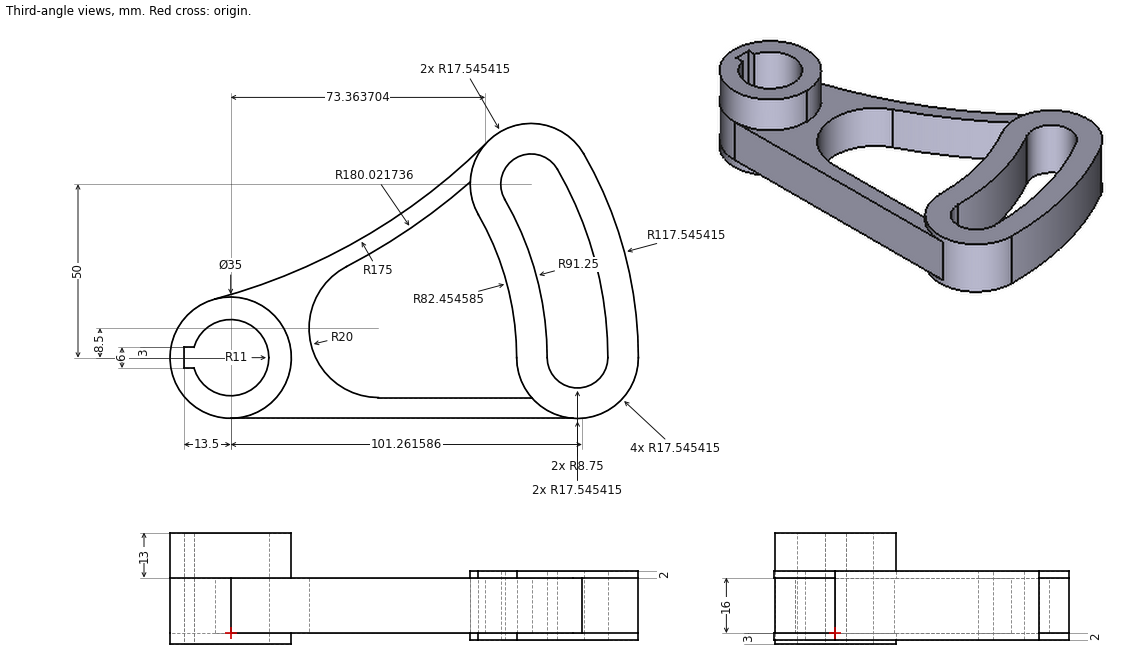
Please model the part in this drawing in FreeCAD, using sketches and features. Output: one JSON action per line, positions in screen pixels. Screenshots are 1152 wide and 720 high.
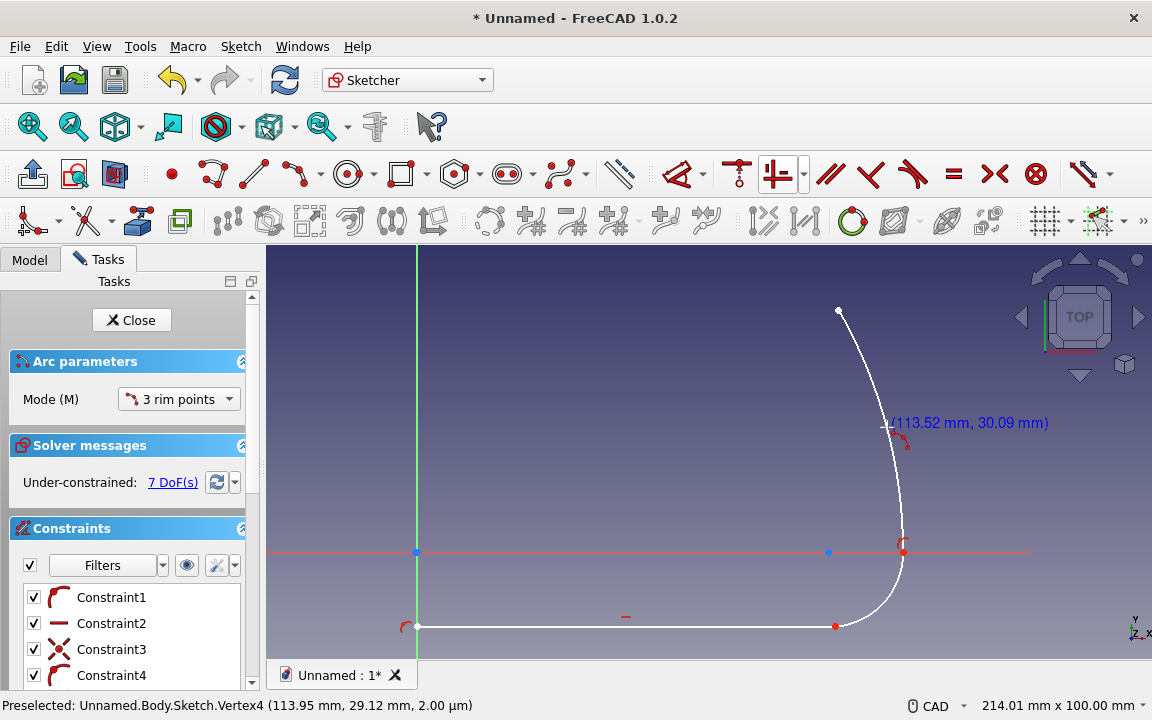
{"action": "left_click", "coordinate": [839, 310]}
{"action": "left_click", "coordinate": [721, 298]}
{"action": "left_click", "coordinate": [783, 273]}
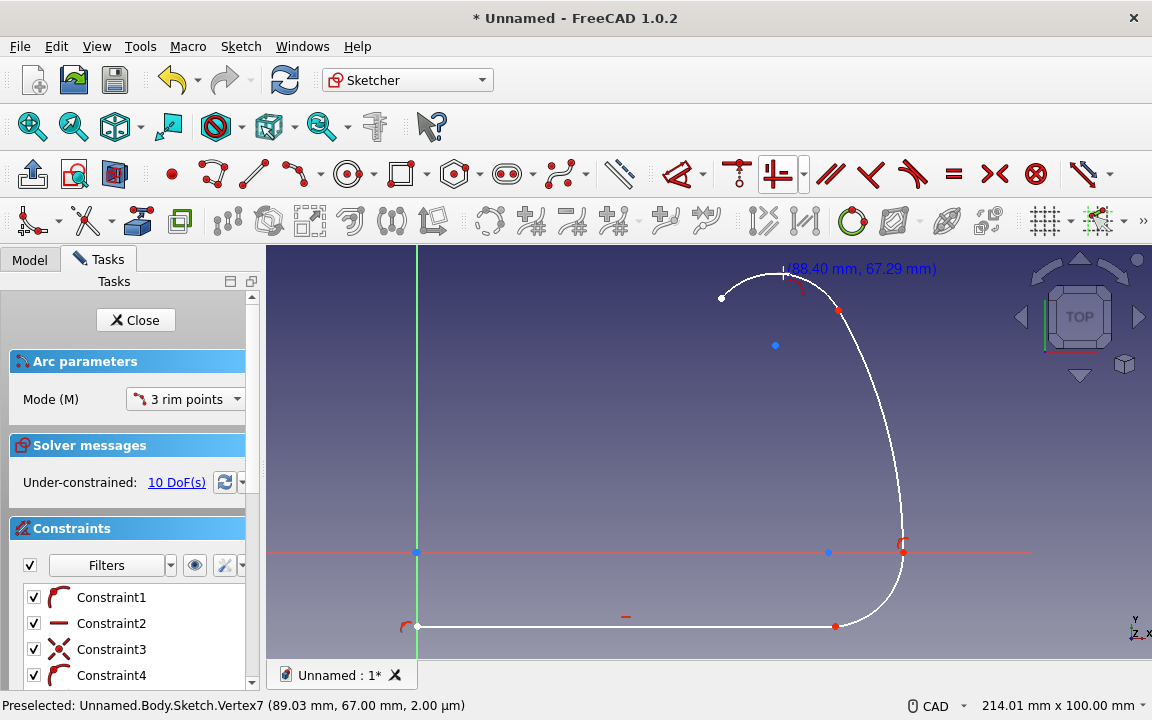
{"action": "left_click", "coordinate": [721, 299]}
{"action": "left_click", "coordinate": [398, 483]}
{"action": "left_click", "coordinate": [572, 411]}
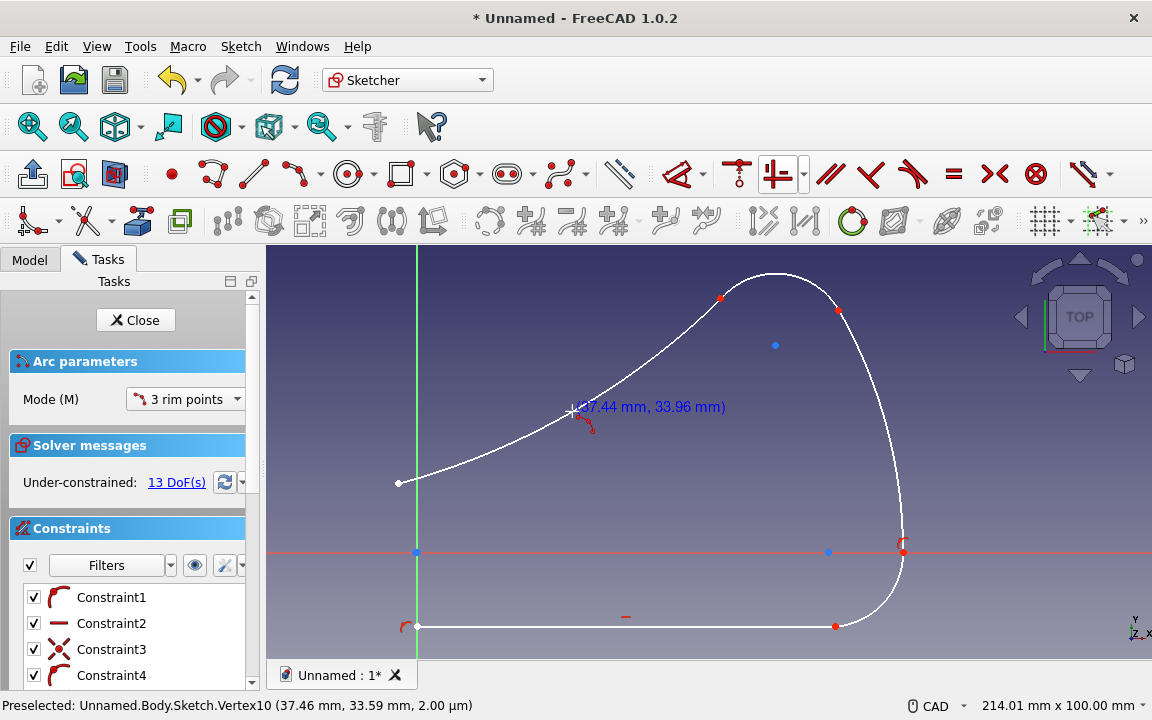
{"action": "left_click", "coordinate": [398, 484]}
{"action": "left_click", "coordinate": [417, 627]}
{"action": "left_click", "coordinate": [351, 582]}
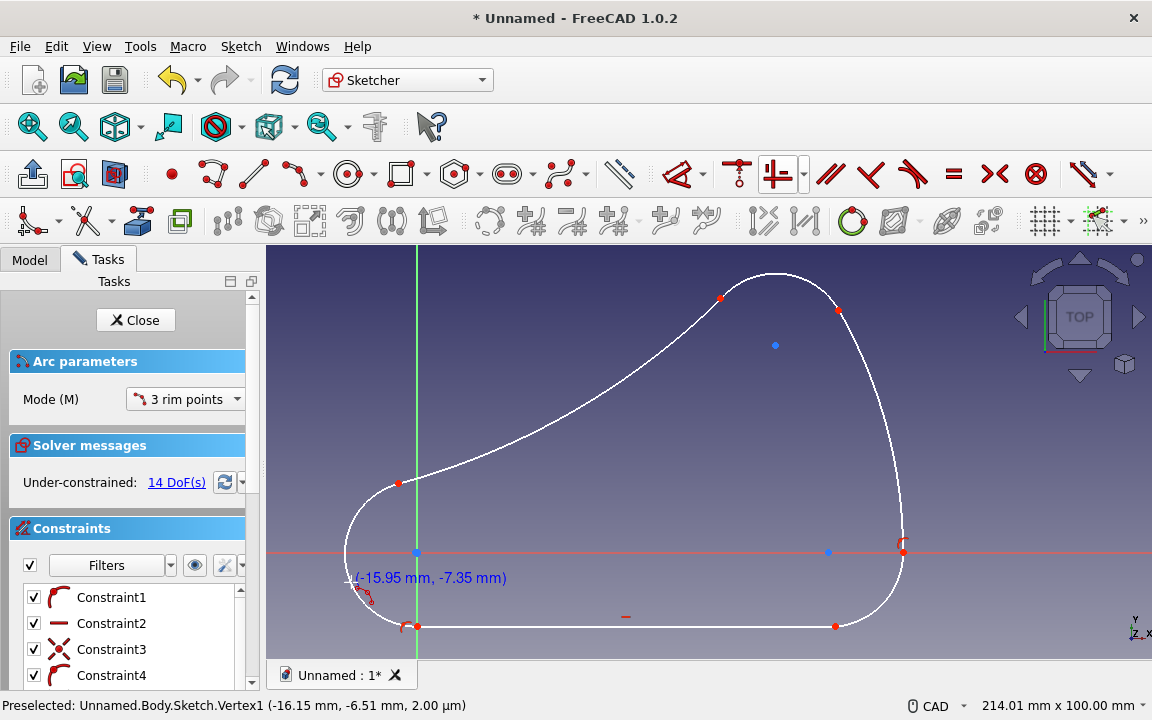
{"action": "left_click", "coordinate": [254, 174]}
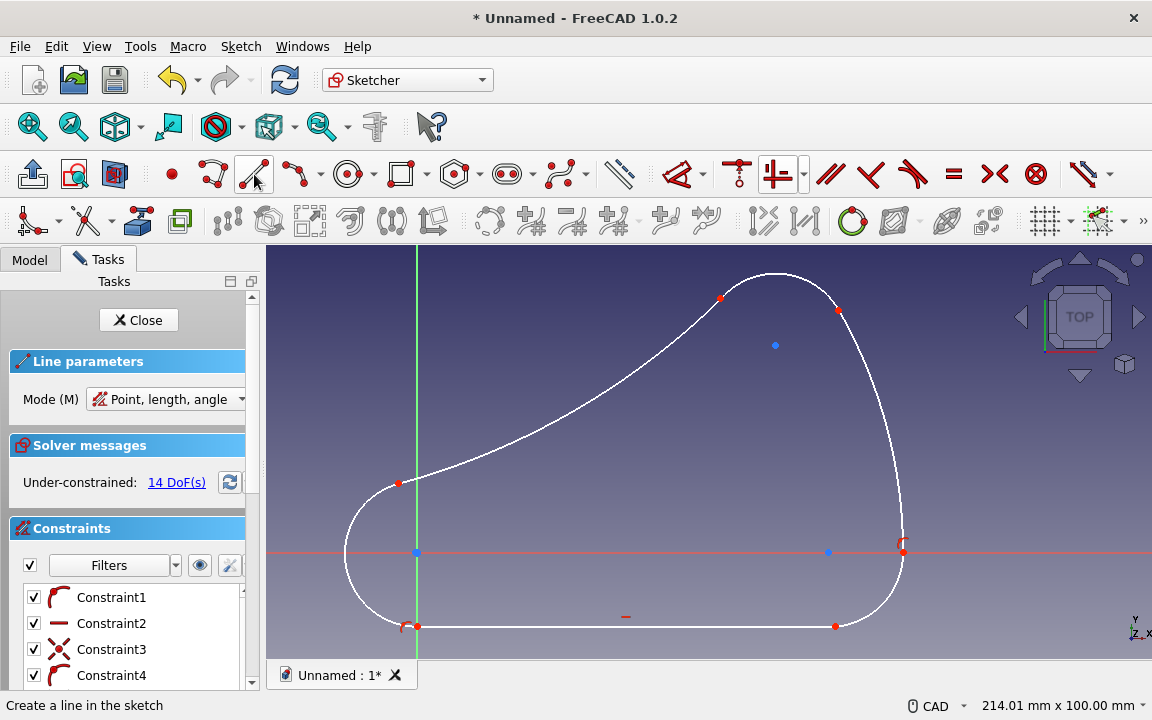
{"action": "left_click", "coordinate": [776, 600]}
{"action": "left_click", "coordinate": [593, 600]}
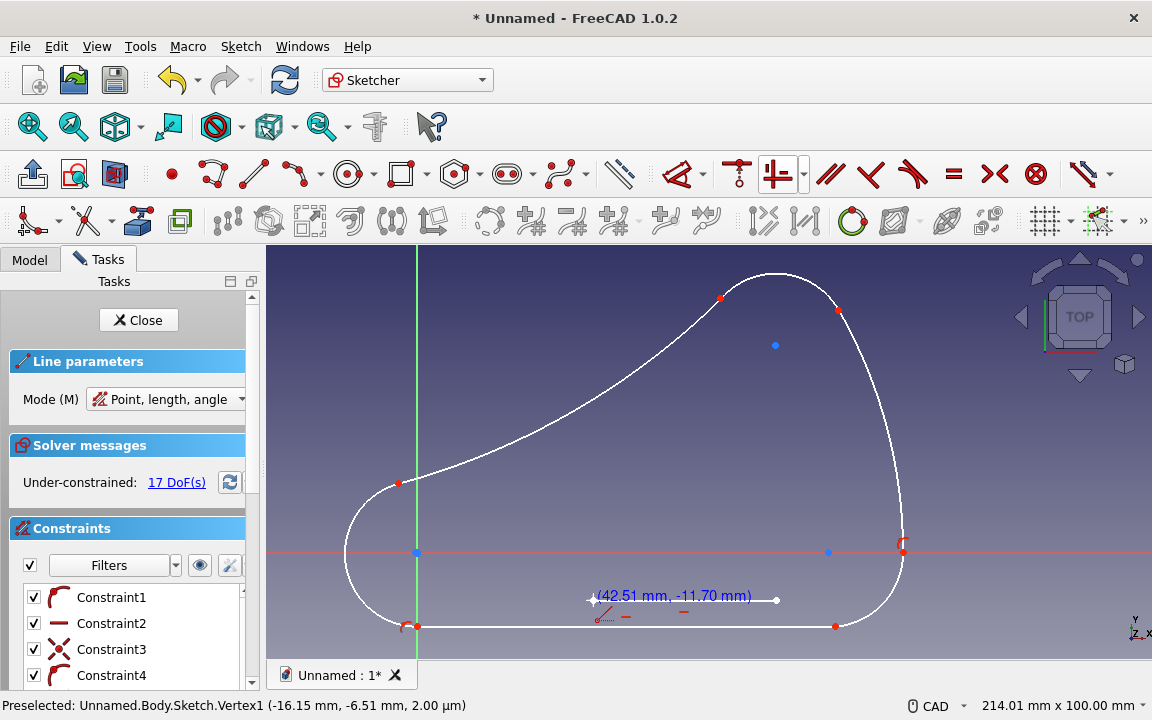
{"action": "left_click", "coordinate": [294, 174]}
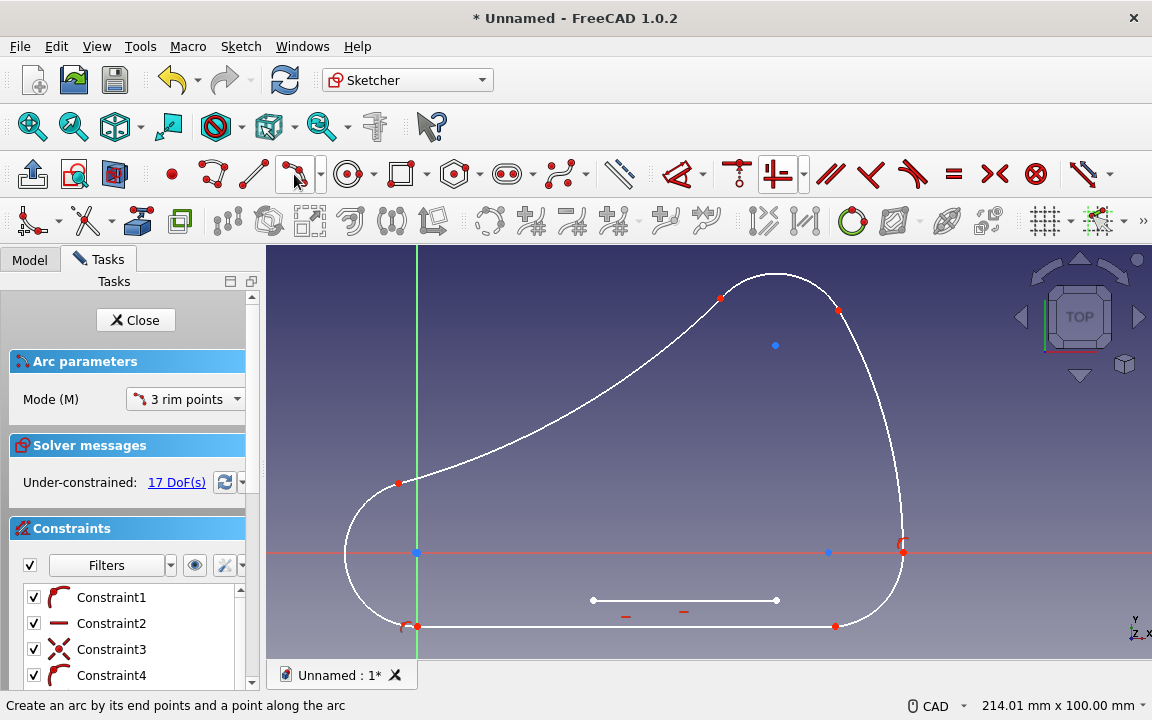
{"action": "left_click", "coordinate": [593, 601]}
{"action": "left_click", "coordinate": [555, 444]}
{"action": "left_click", "coordinate": [511, 515]}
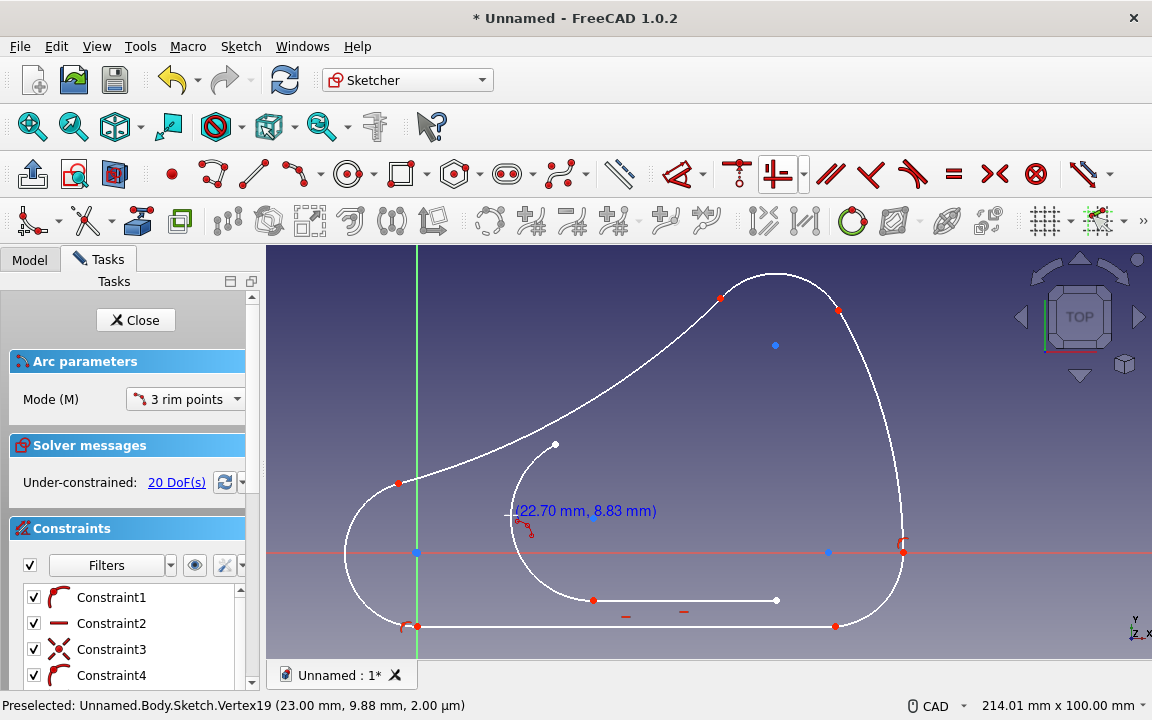
{"action": "left_click", "coordinate": [555, 445]}
{"action": "left_click", "coordinate": [703, 343]}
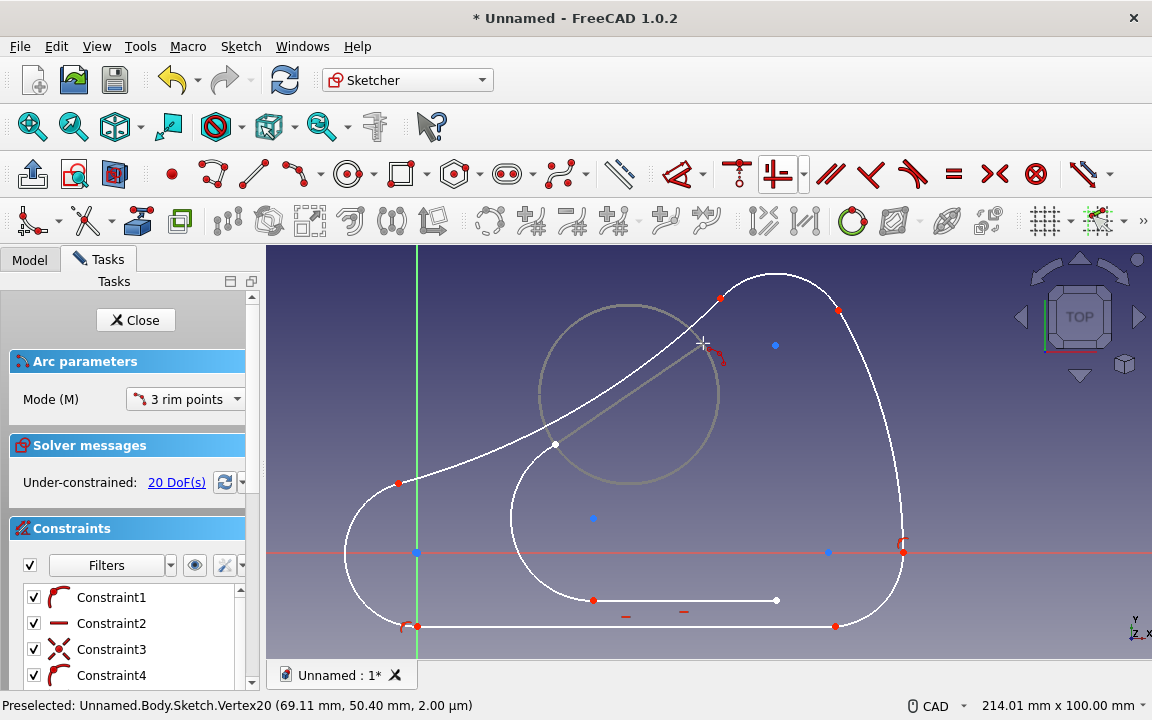
{"action": "scroll", "coordinate": [632, 398], "scroll_direction": "up", "scroll_amount": 6}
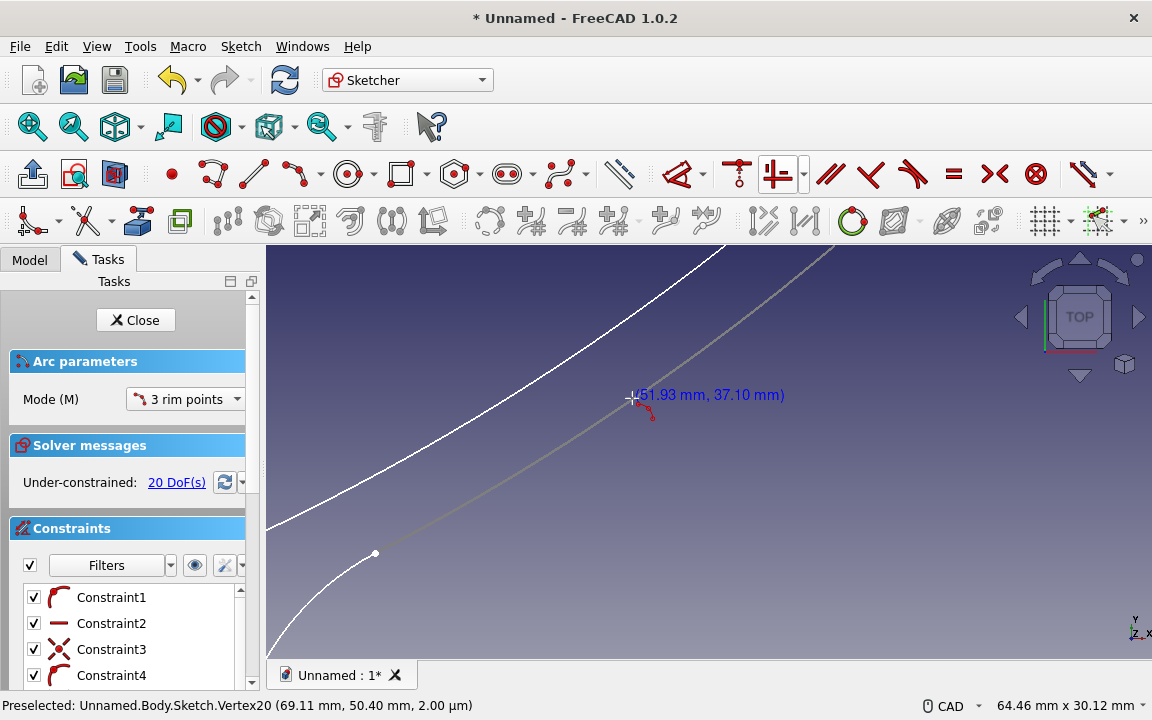
{"action": "left_click", "coordinate": [631, 397]}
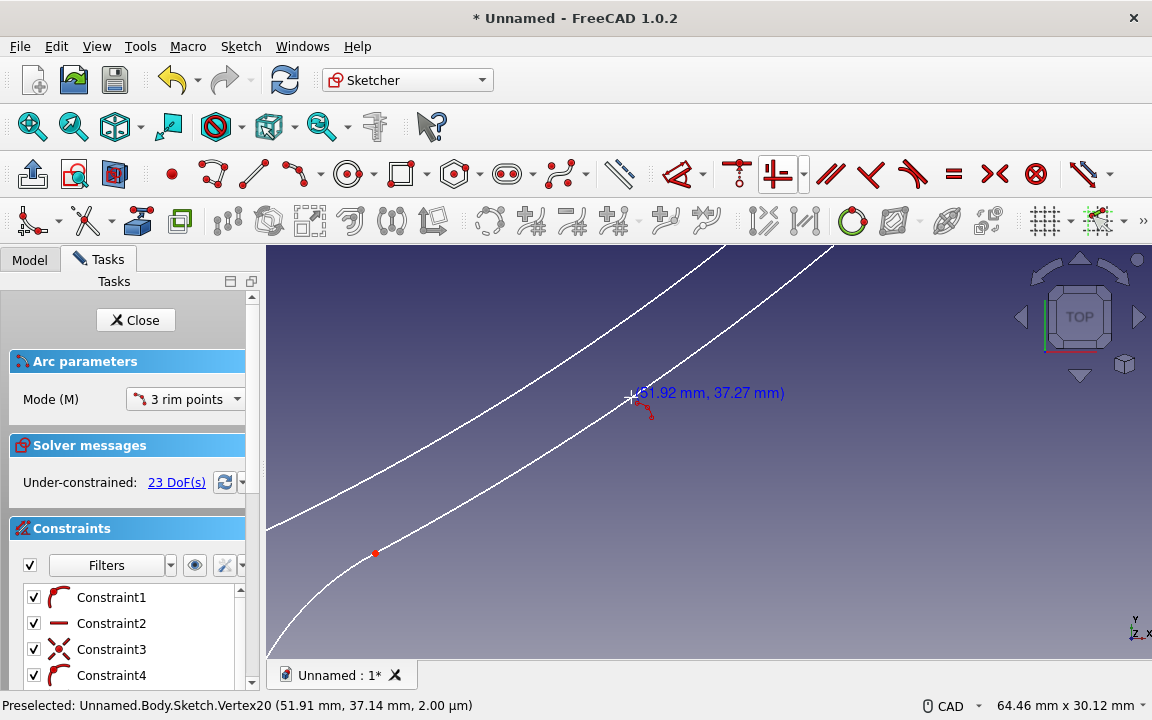
{"action": "scroll", "coordinate": [649, 423], "scroll_direction": "down", "scroll_amount": 8}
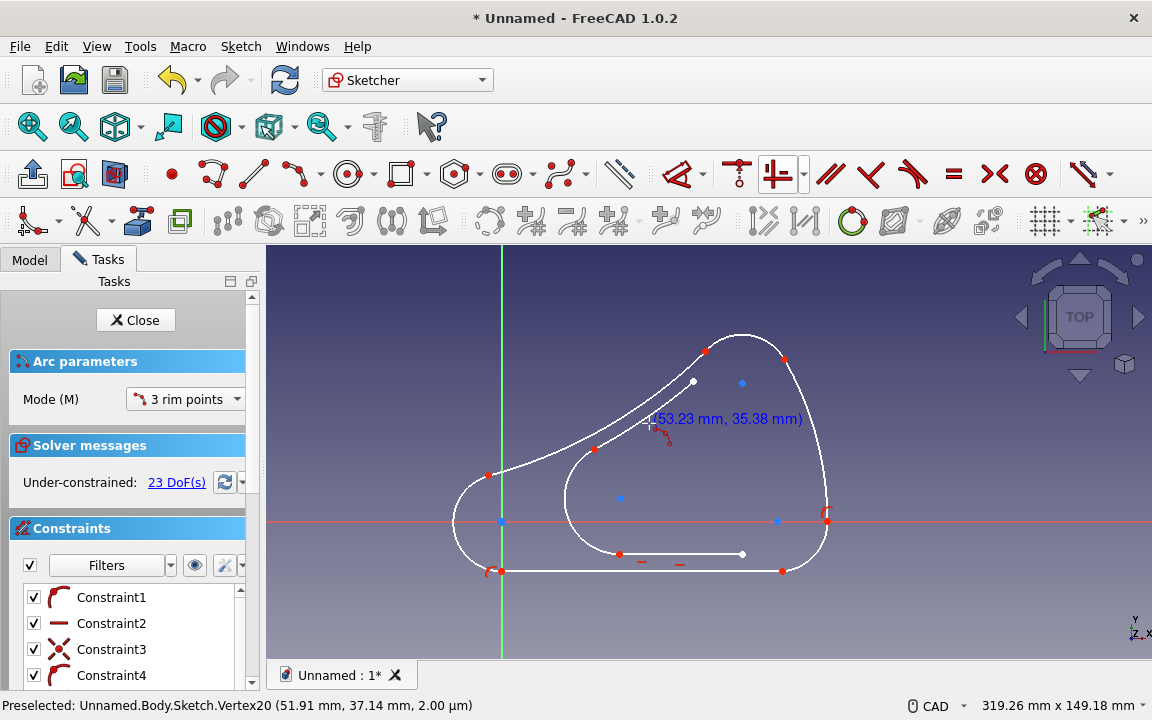
{"action": "left_click", "coordinate": [693, 382]}
{"action": "left_click", "coordinate": [700, 407]}